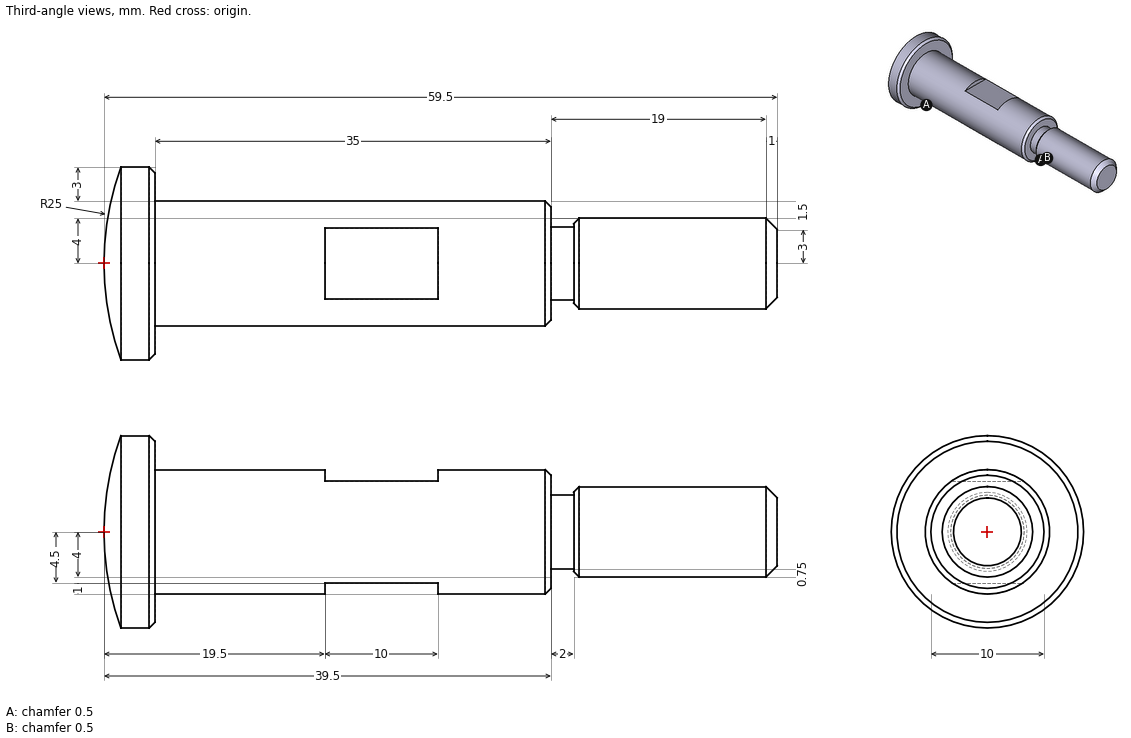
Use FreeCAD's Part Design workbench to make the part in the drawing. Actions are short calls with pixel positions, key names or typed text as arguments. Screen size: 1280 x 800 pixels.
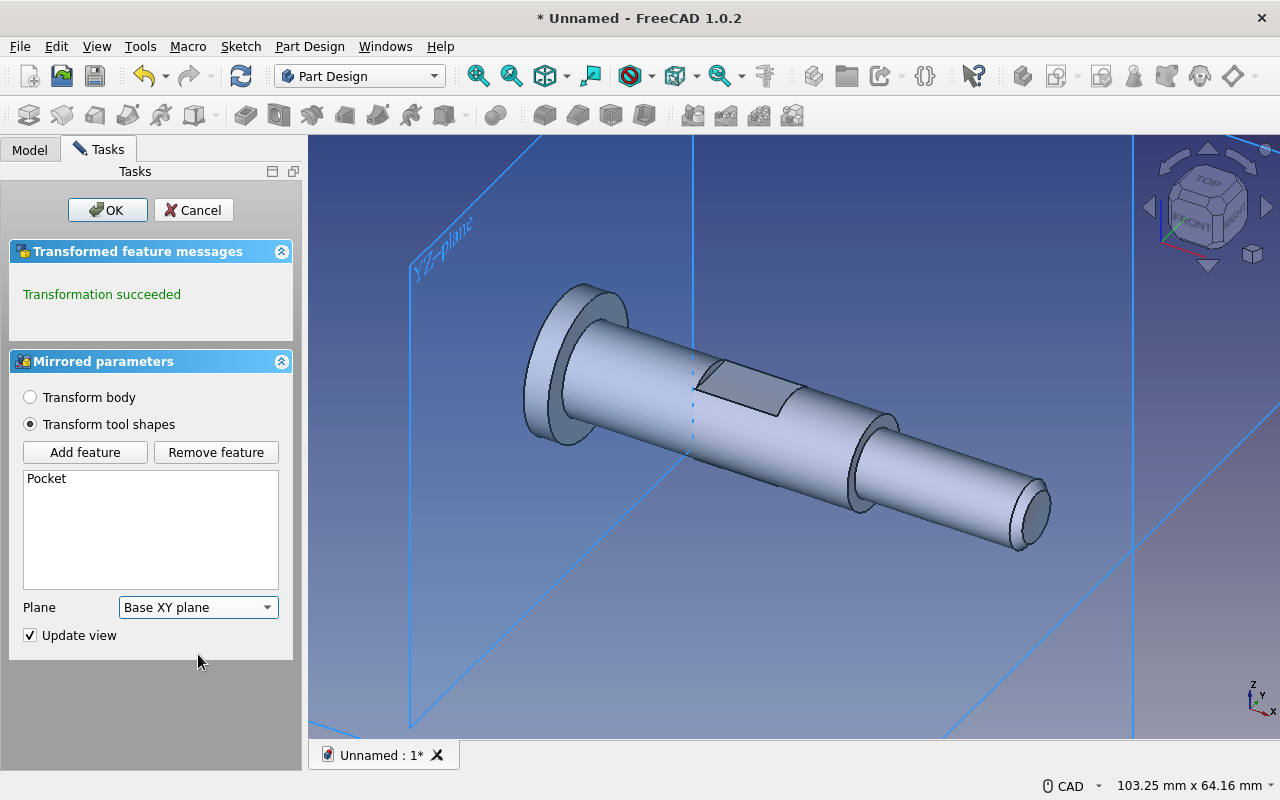
click(108, 210)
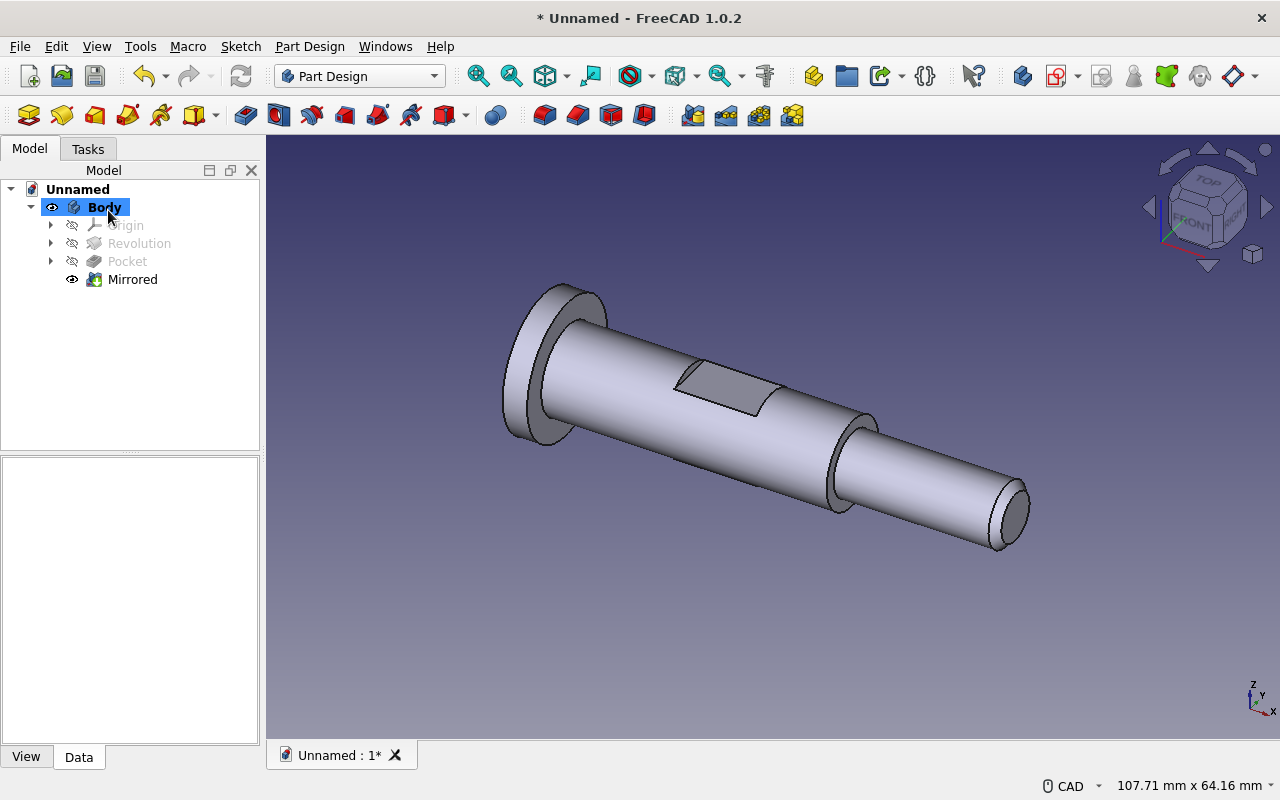
click(527, 408)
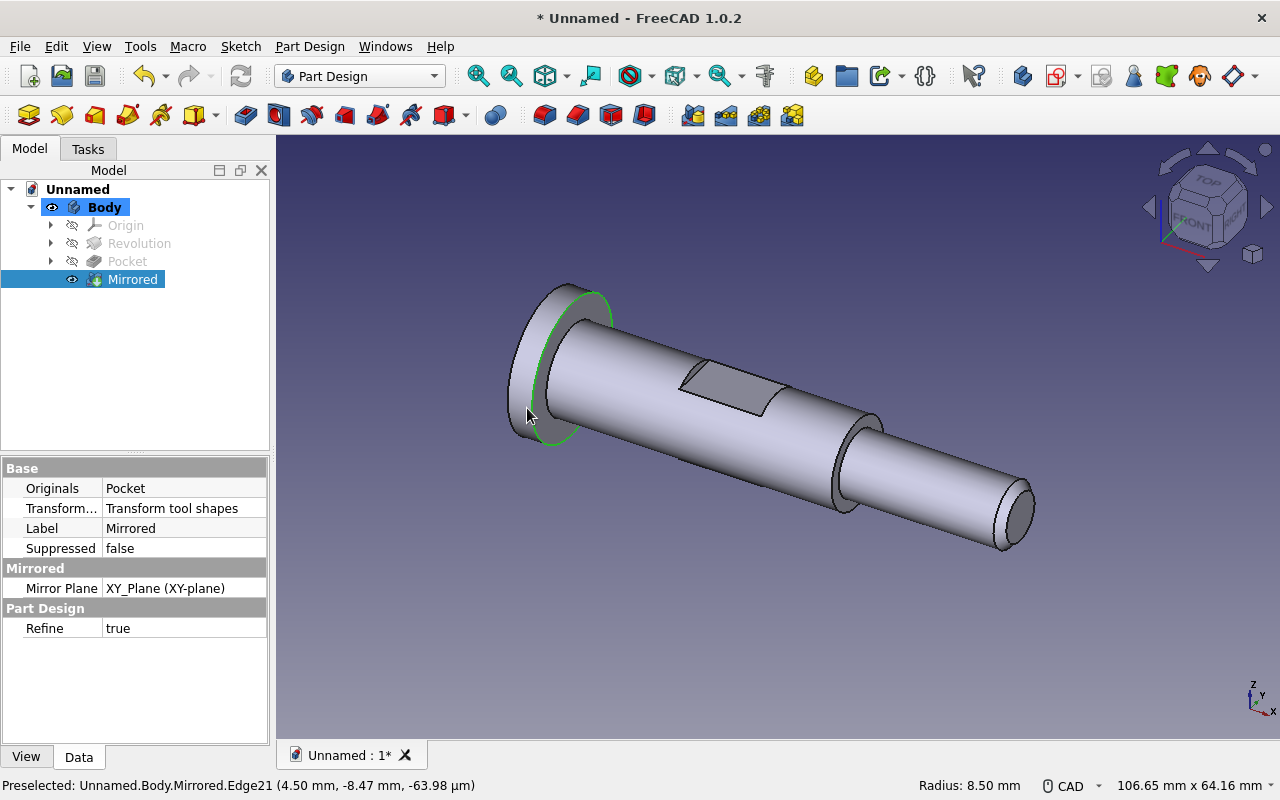
click(832, 488, ctrl)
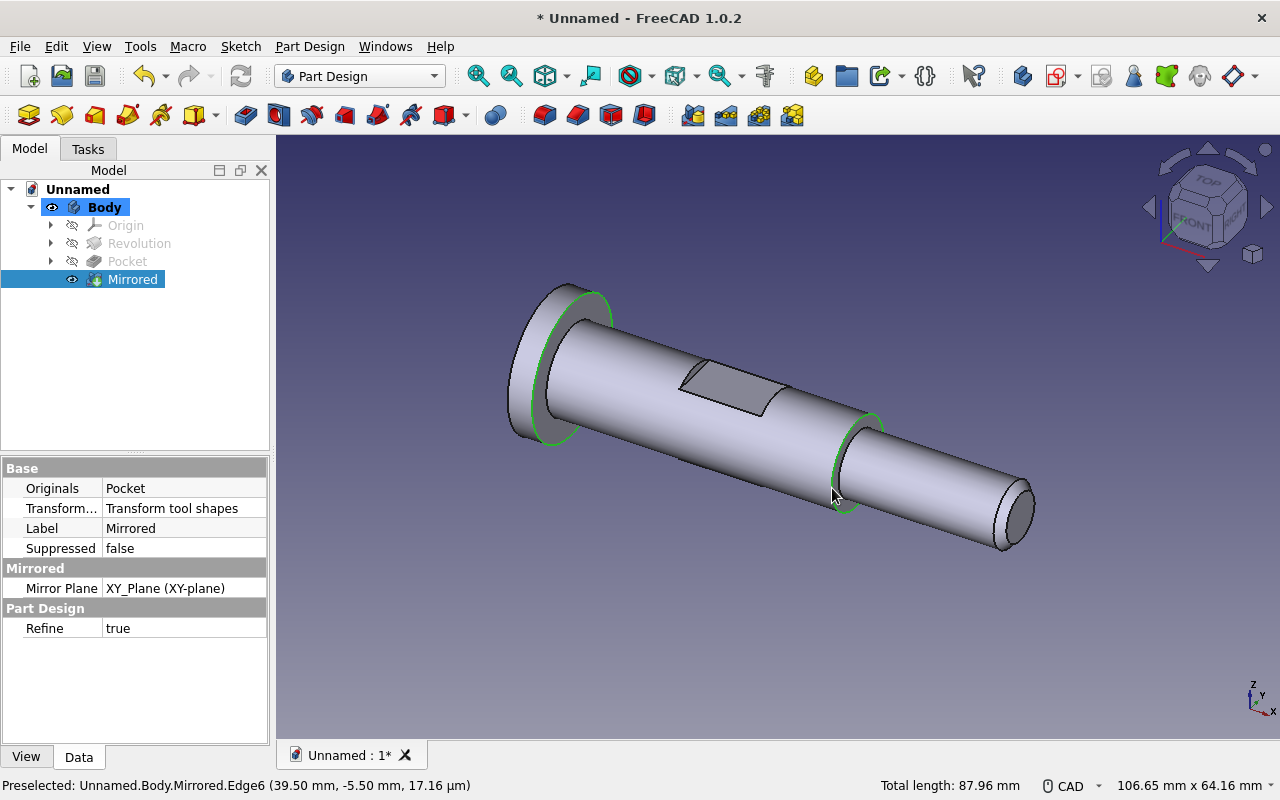
click(578, 116)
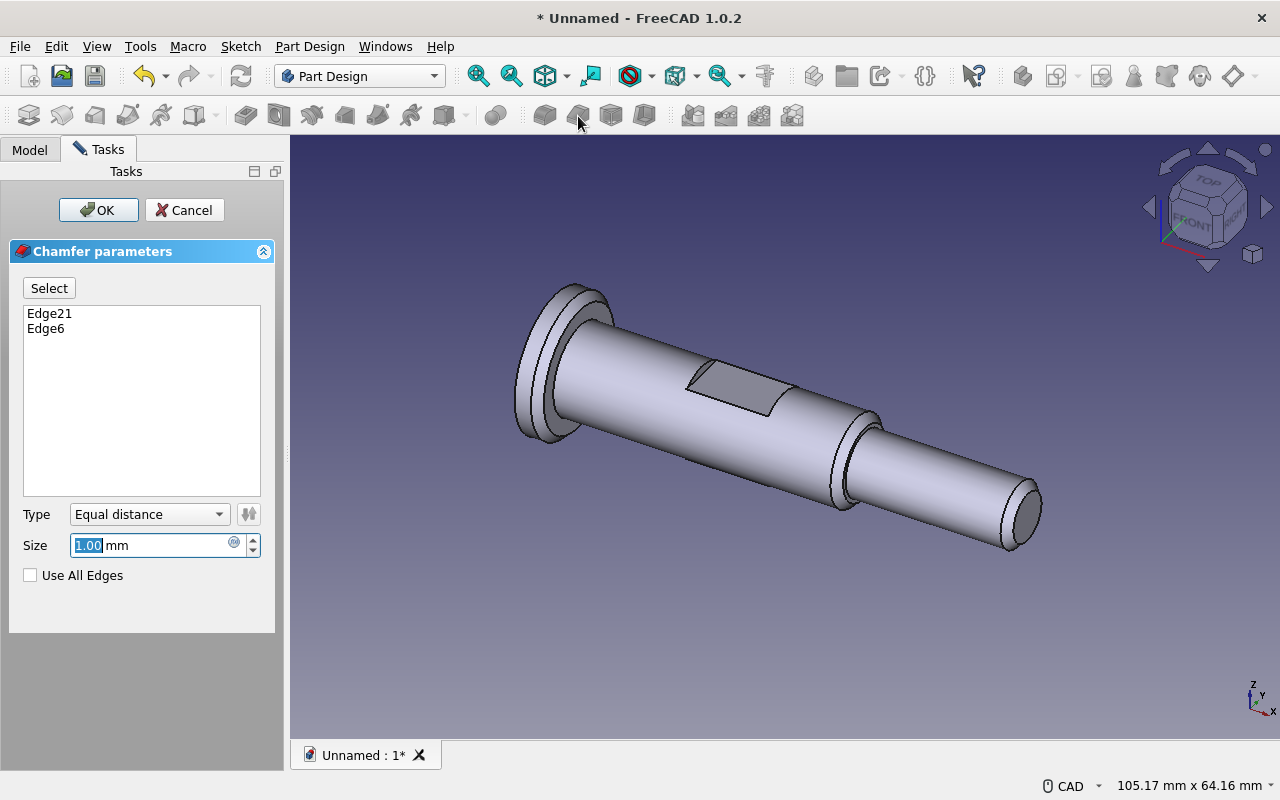
text(0.5)
key(Tab)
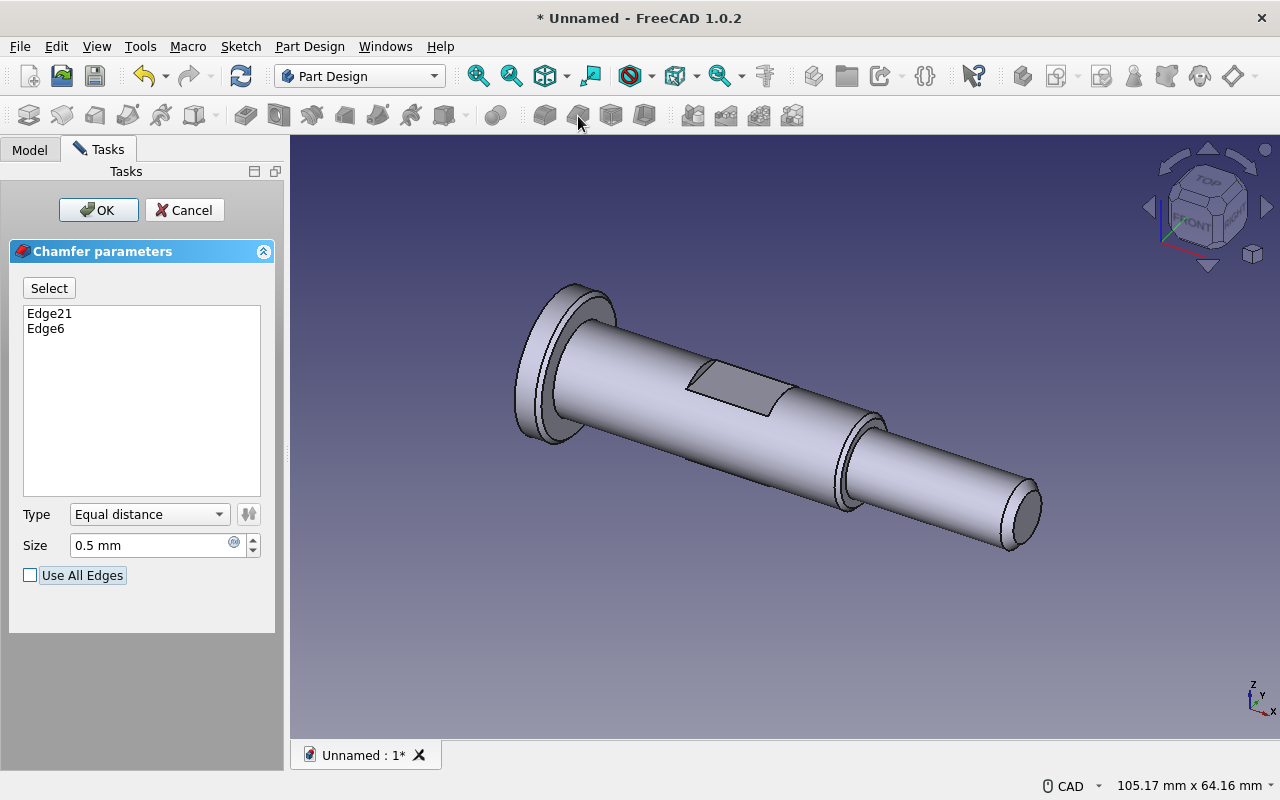
click(99, 210)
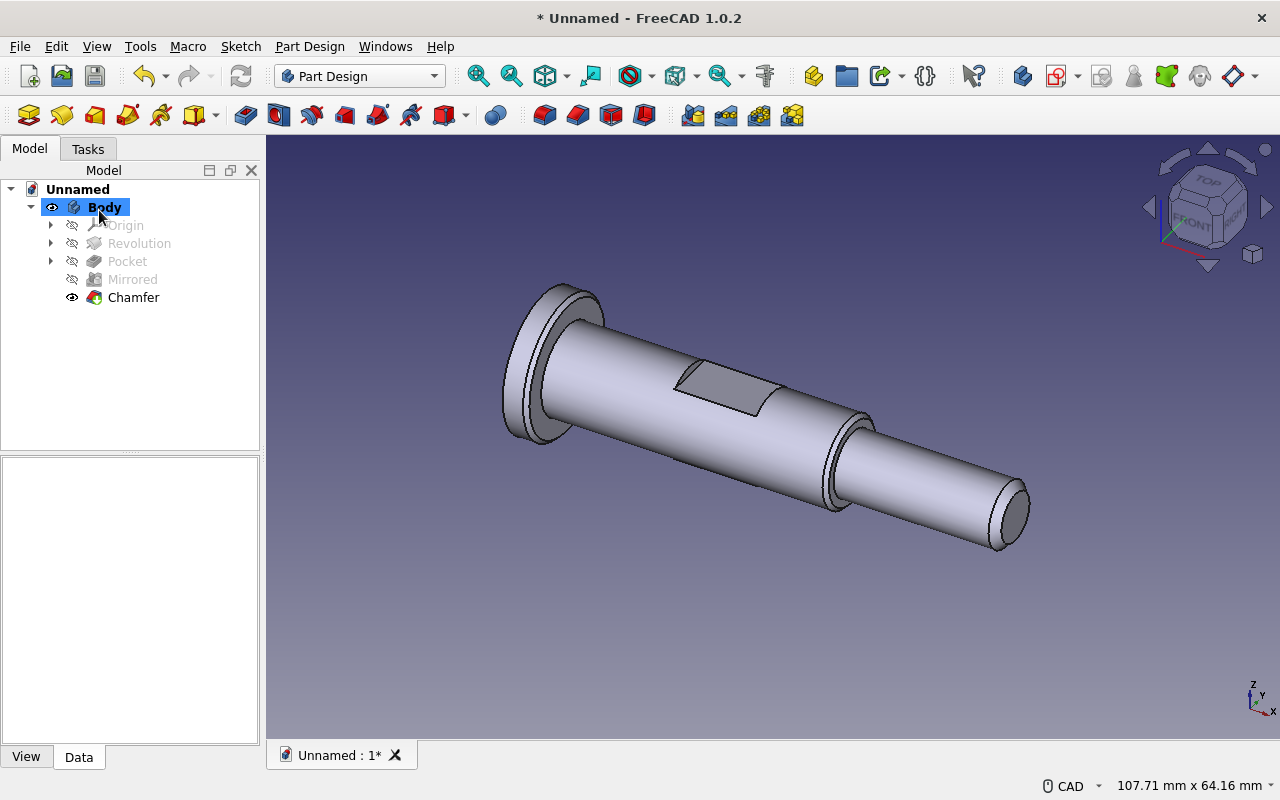
click(1056, 76)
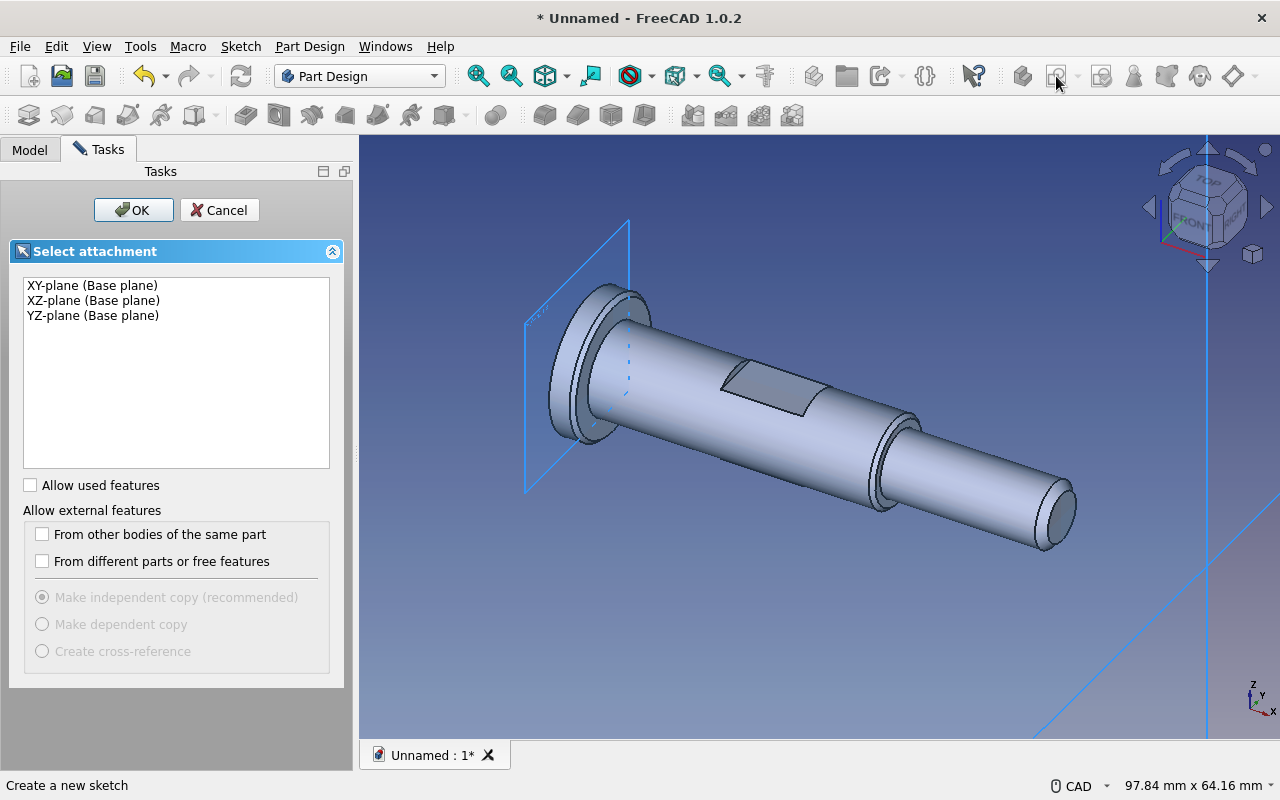
click(84, 300)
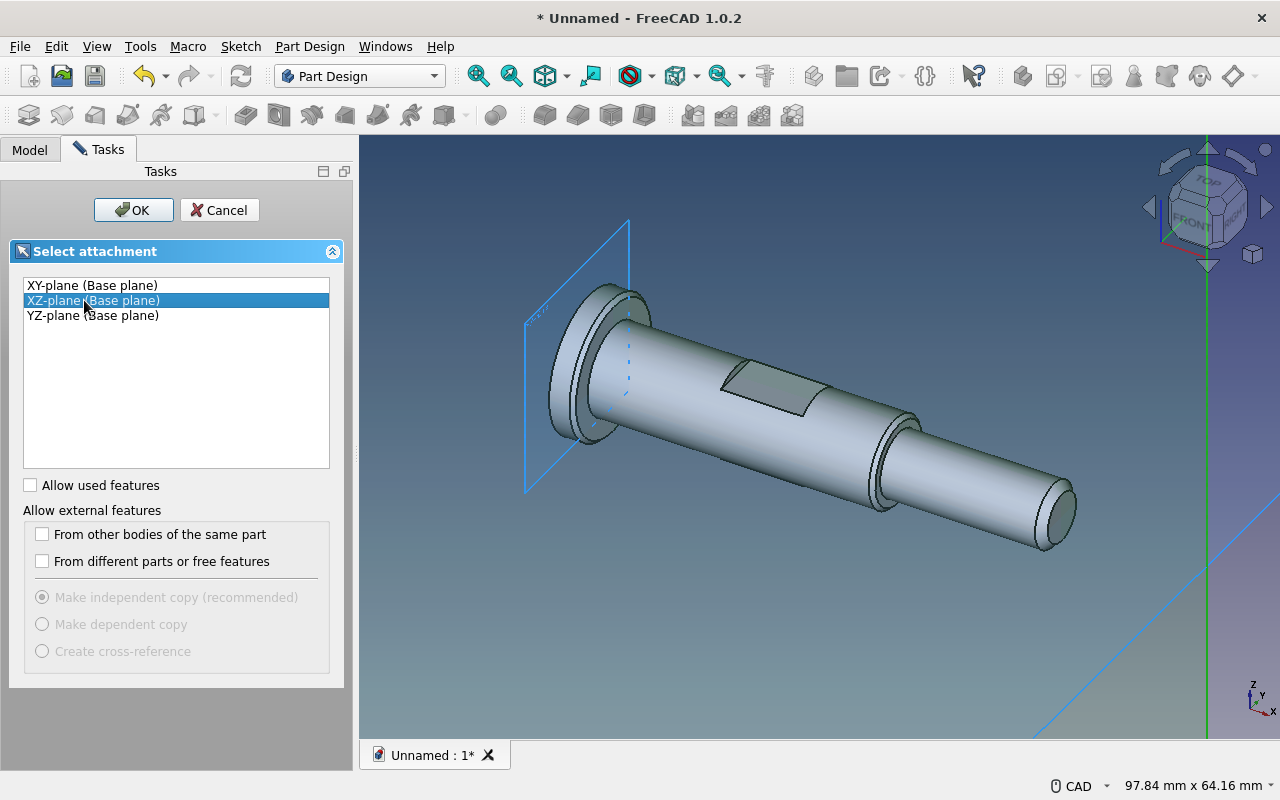
click(134, 210)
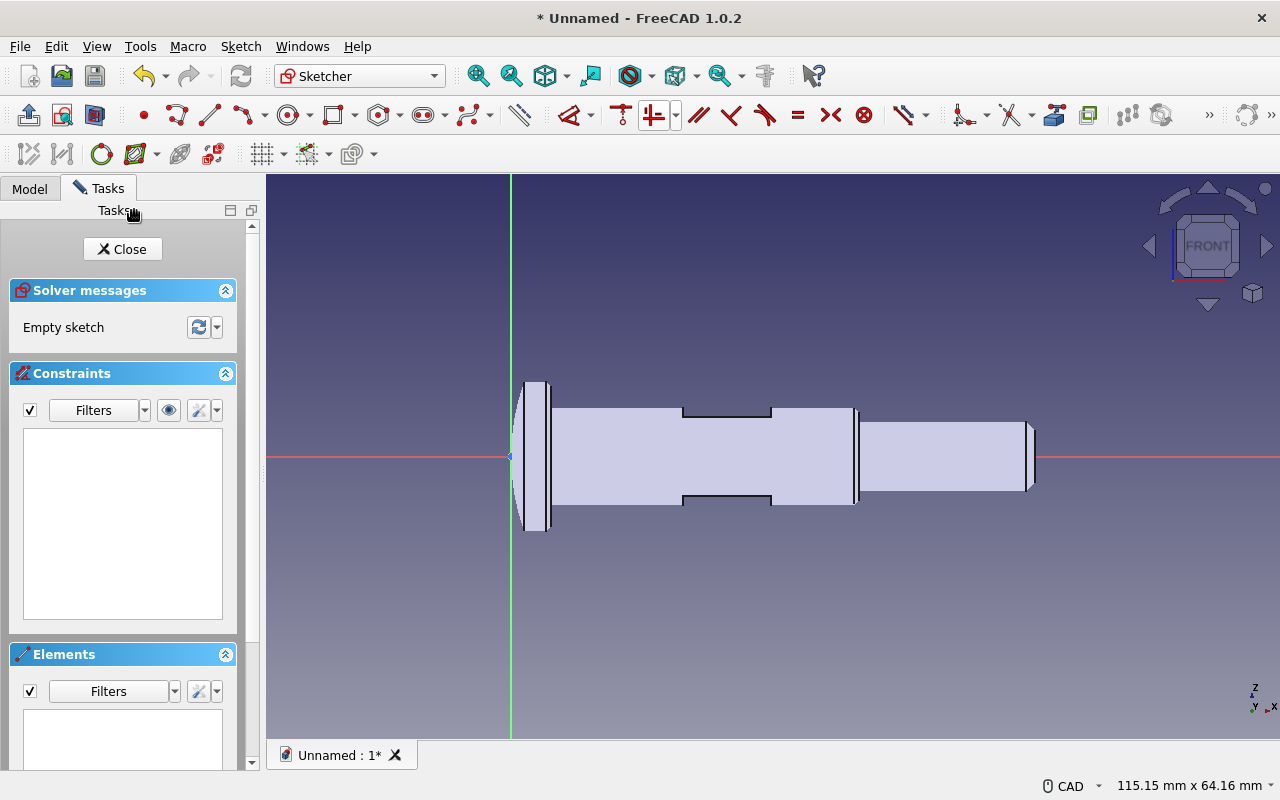
click(95, 116)